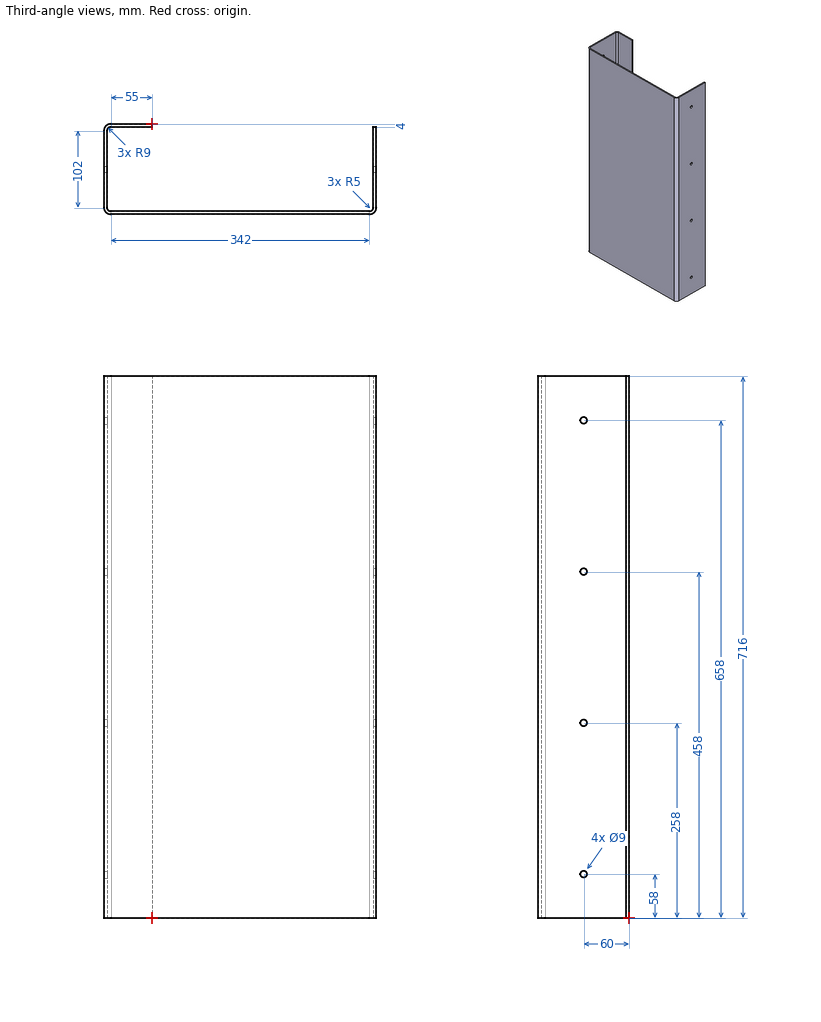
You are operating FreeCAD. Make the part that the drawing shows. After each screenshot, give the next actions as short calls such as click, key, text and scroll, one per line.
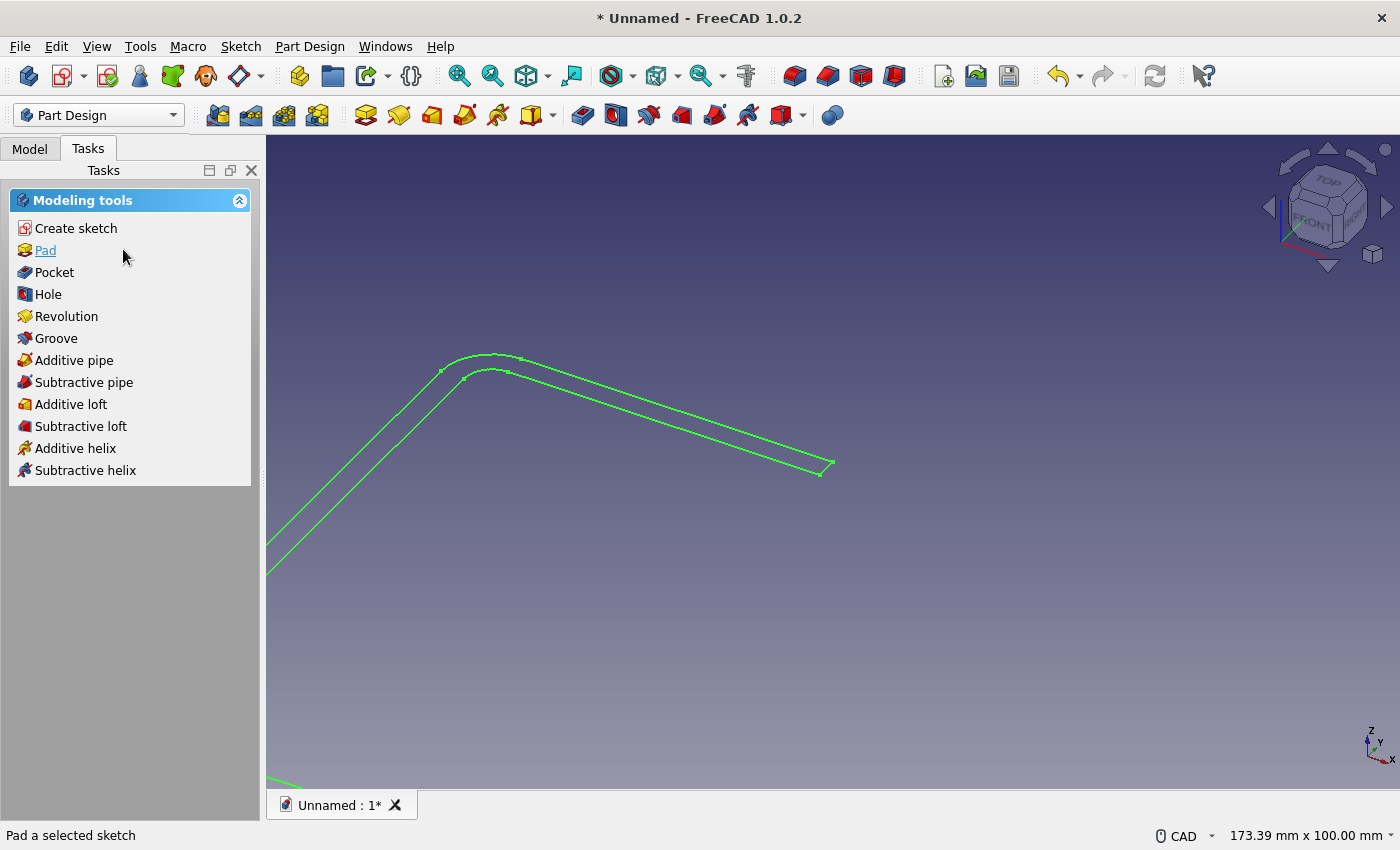
click(366, 116)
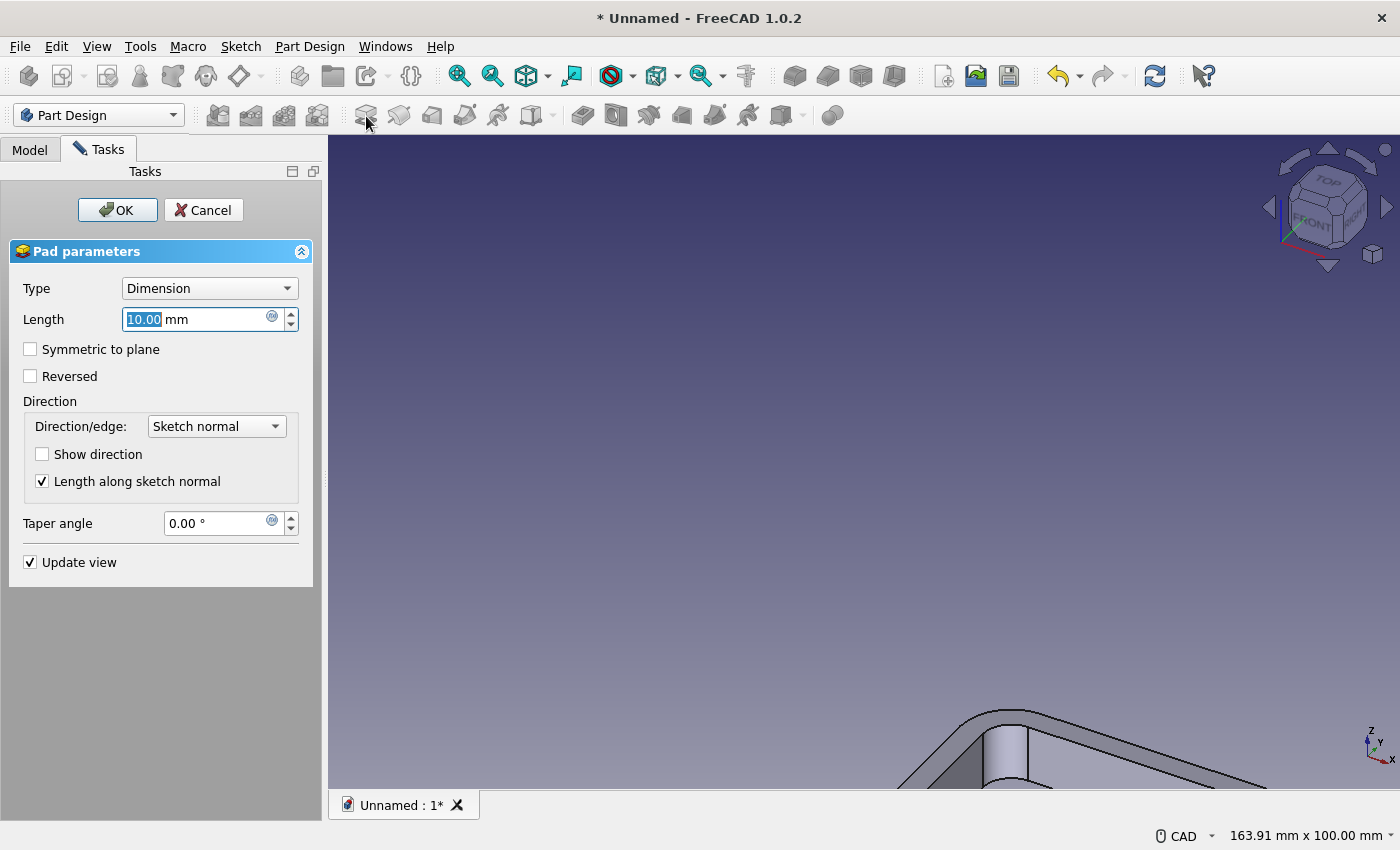
text(716)
key(Tab)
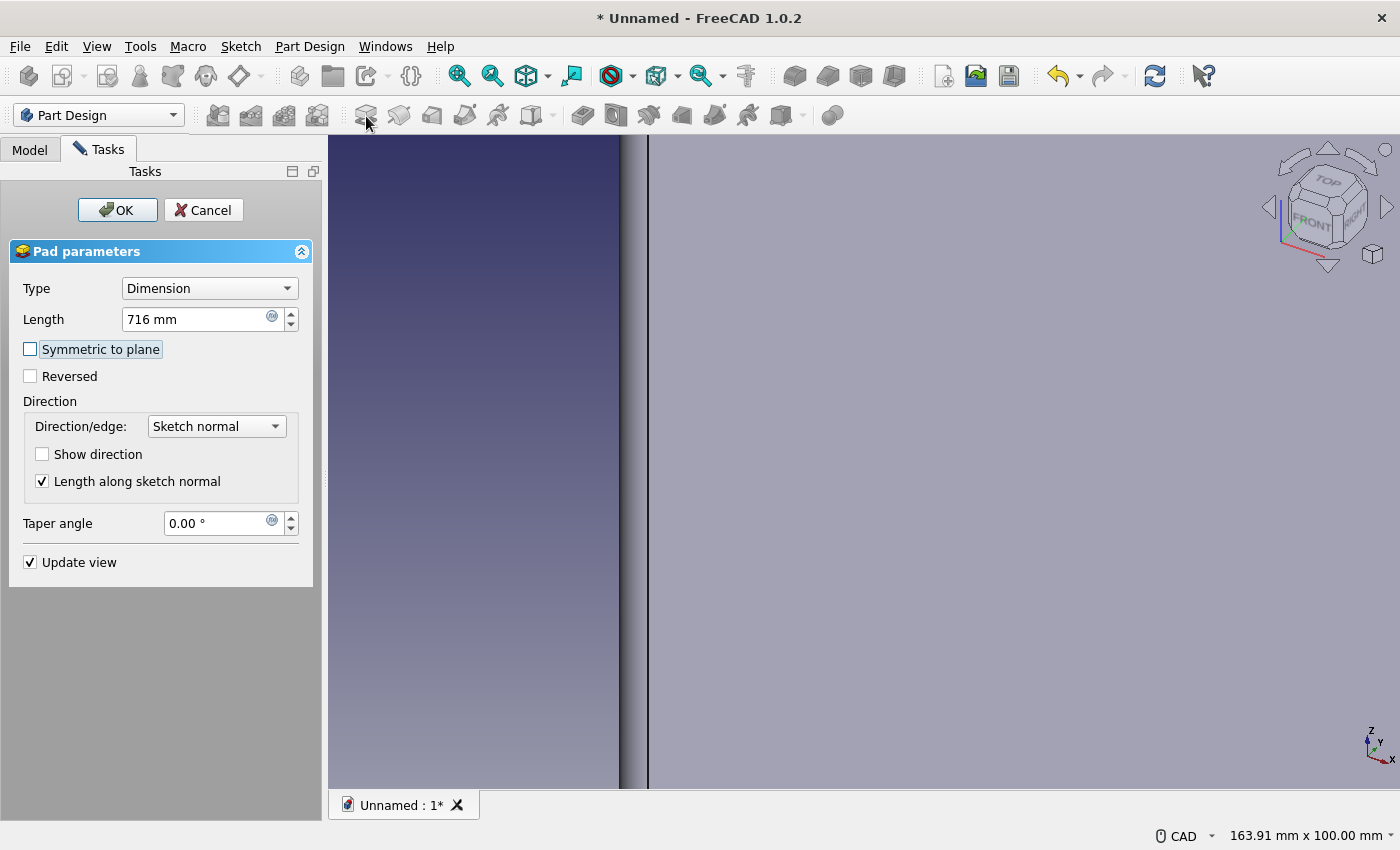
click(118, 210)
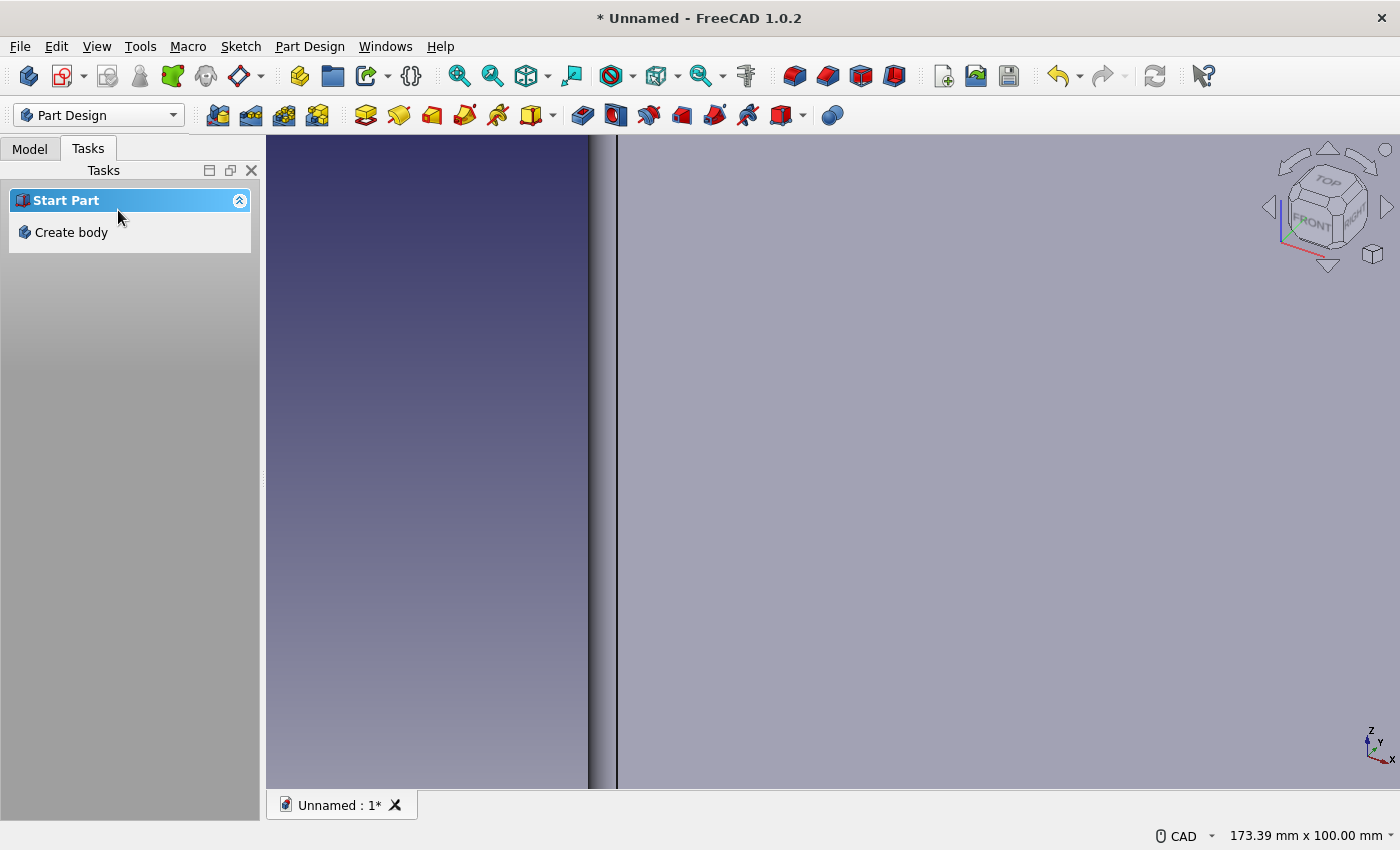
click(460, 76)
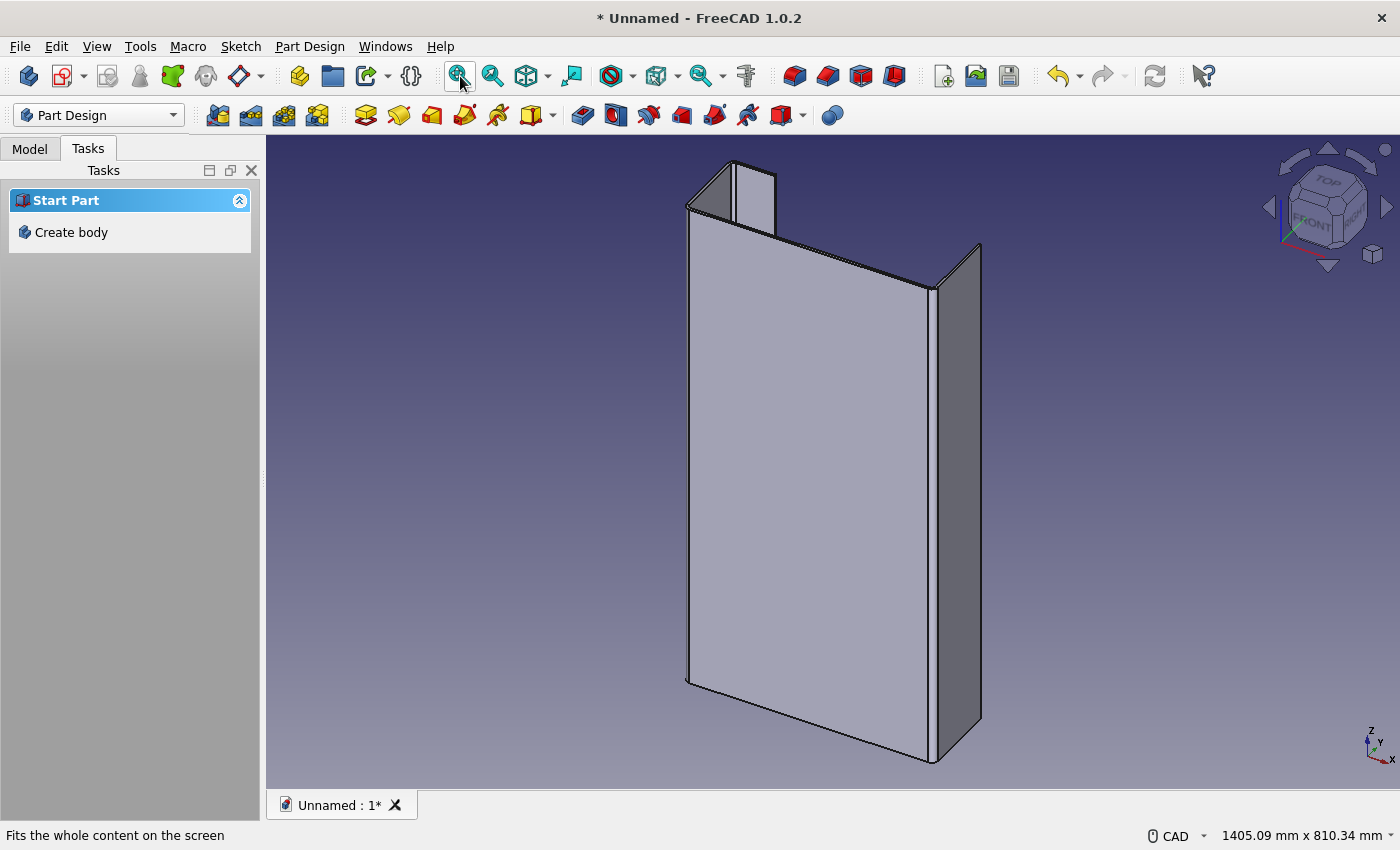
key(6)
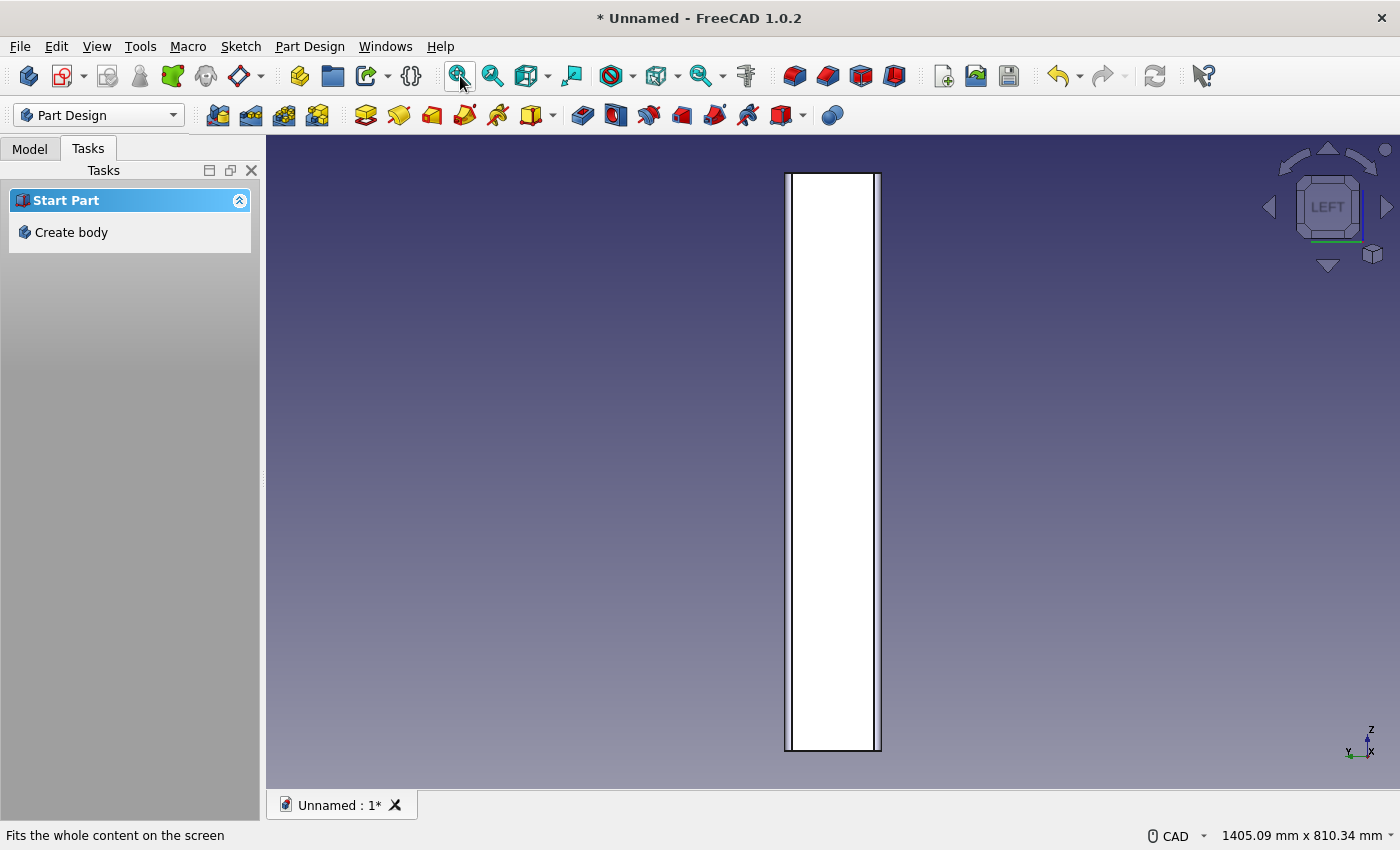
click(833, 213)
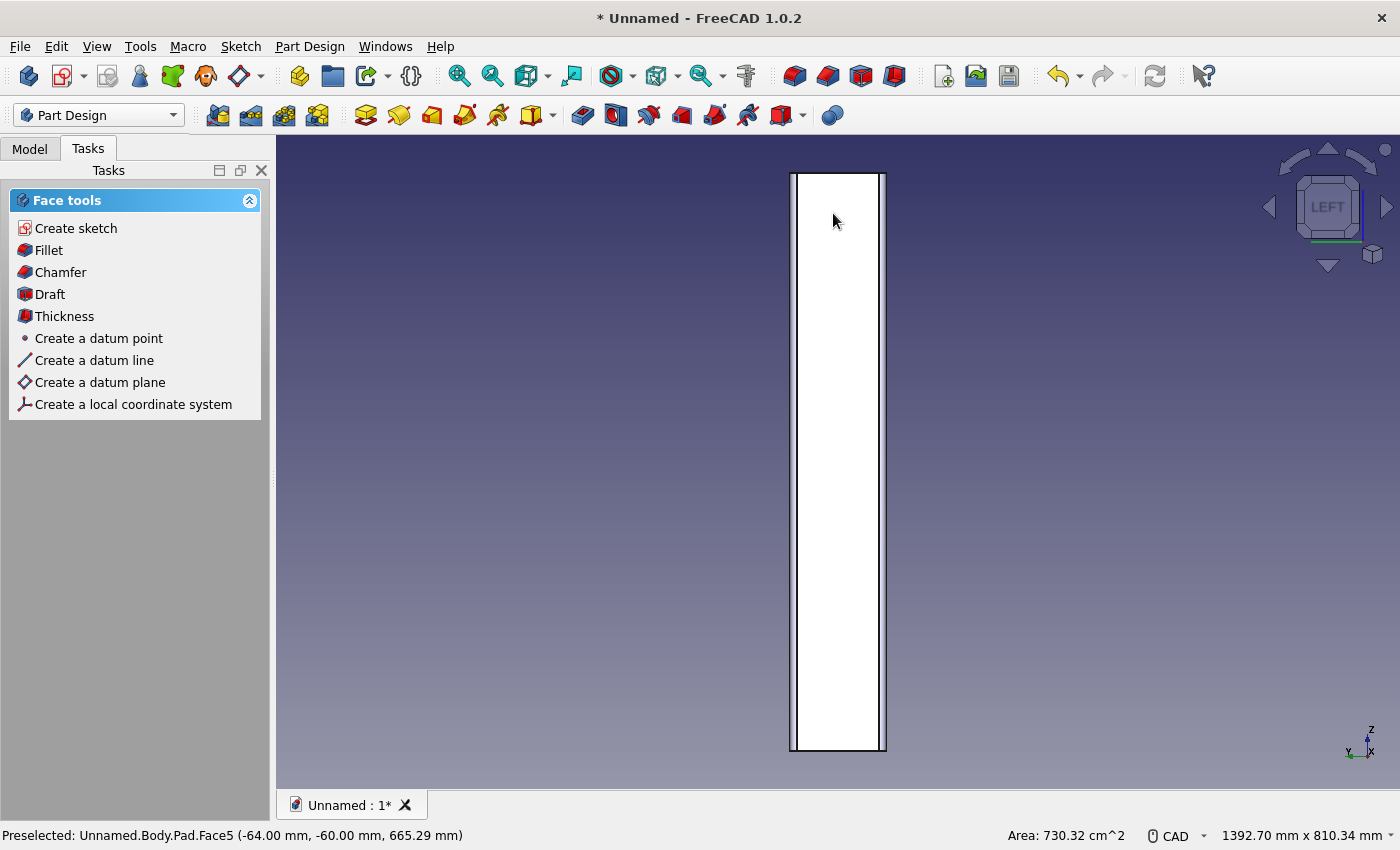
click(62, 76)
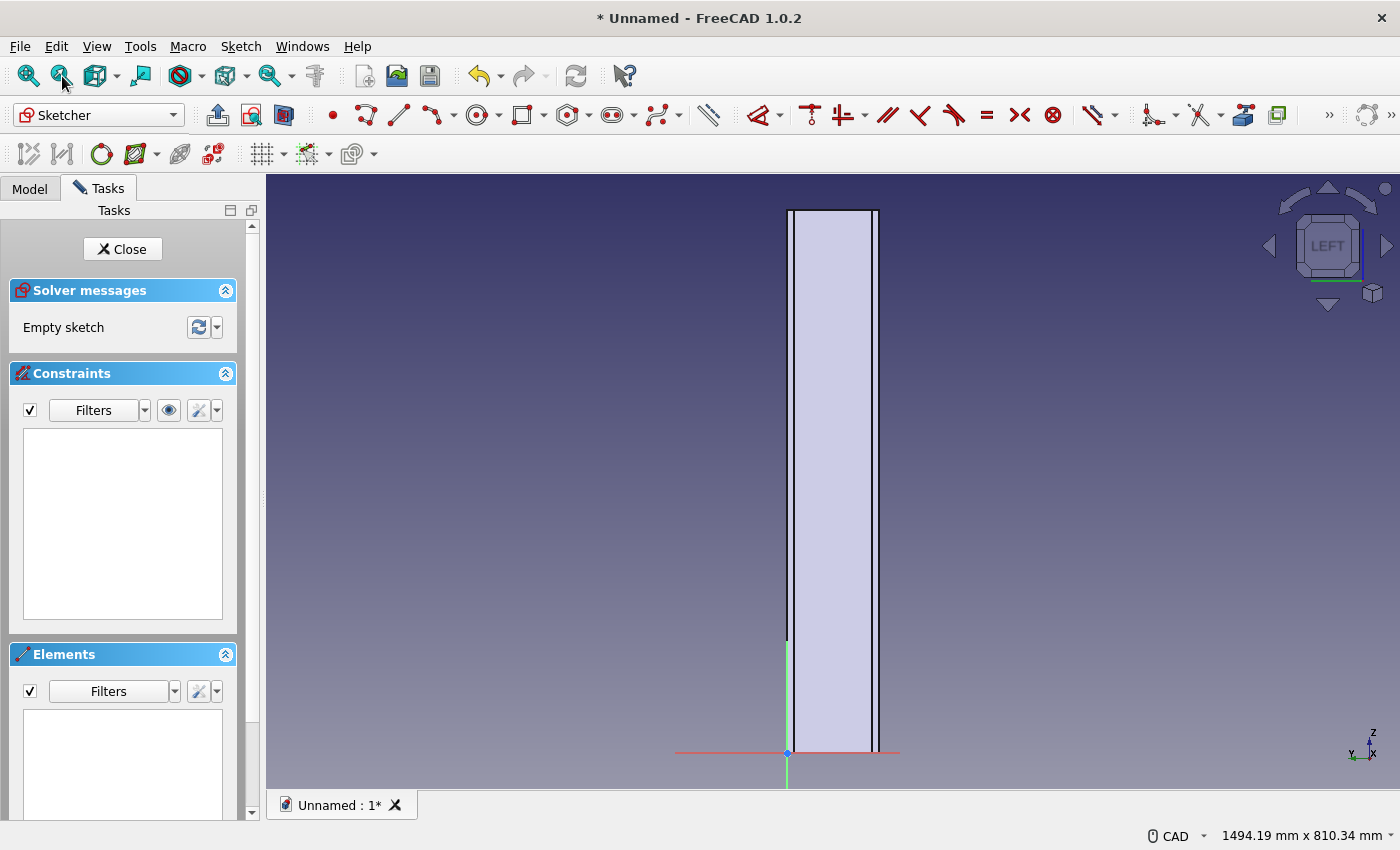
scroll(550, 390, down, 1)